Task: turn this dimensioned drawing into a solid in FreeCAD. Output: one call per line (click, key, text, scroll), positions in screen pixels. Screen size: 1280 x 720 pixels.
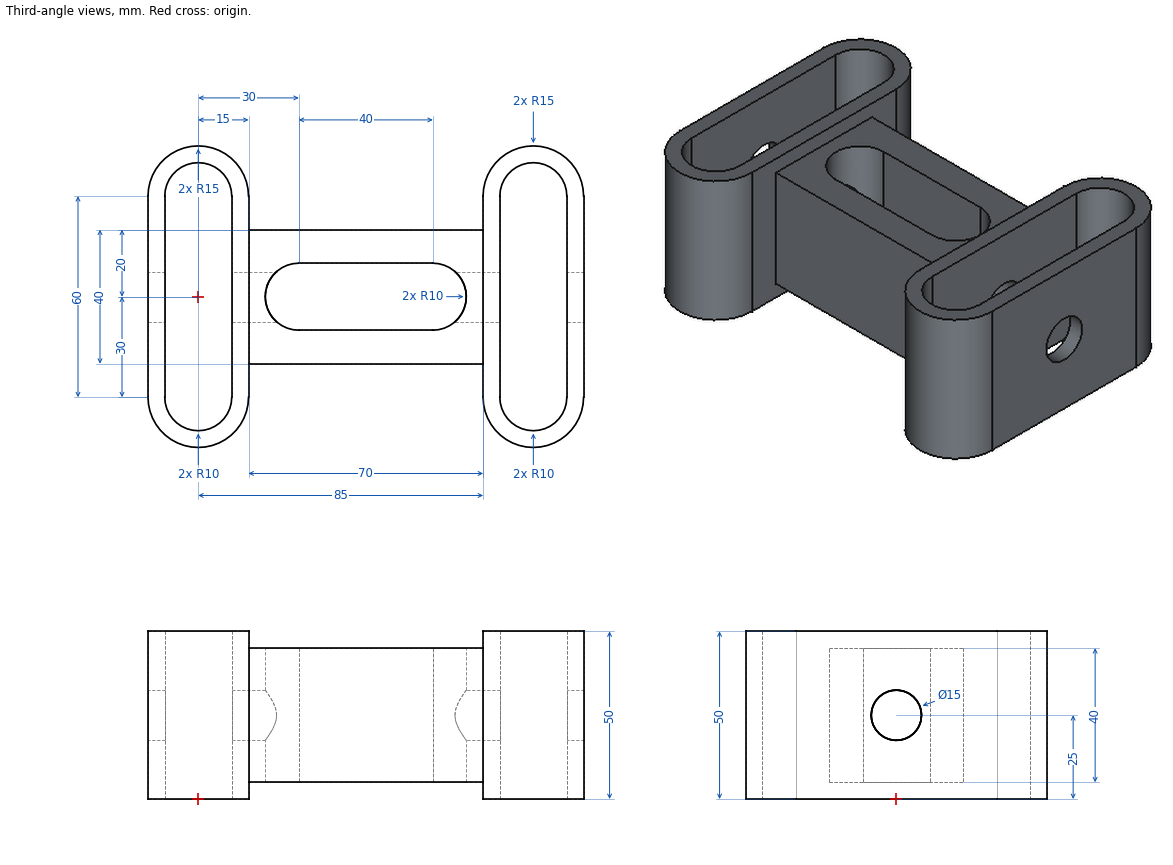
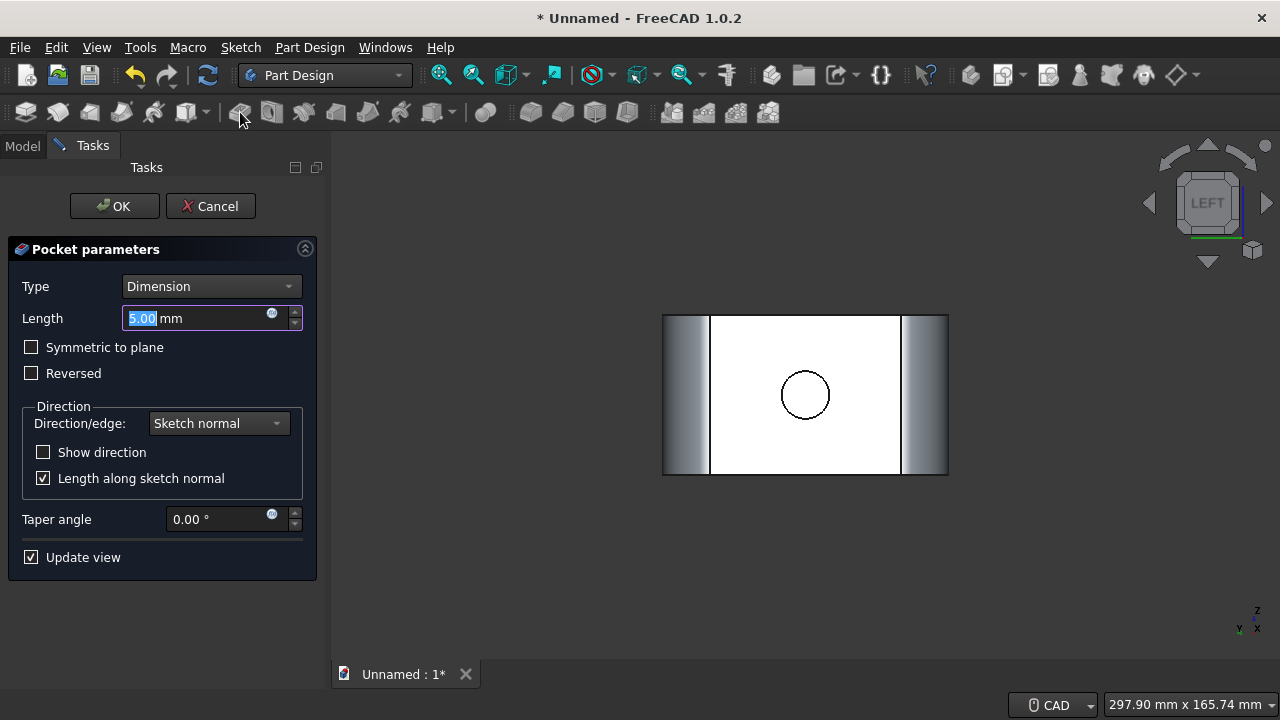
click(212, 286)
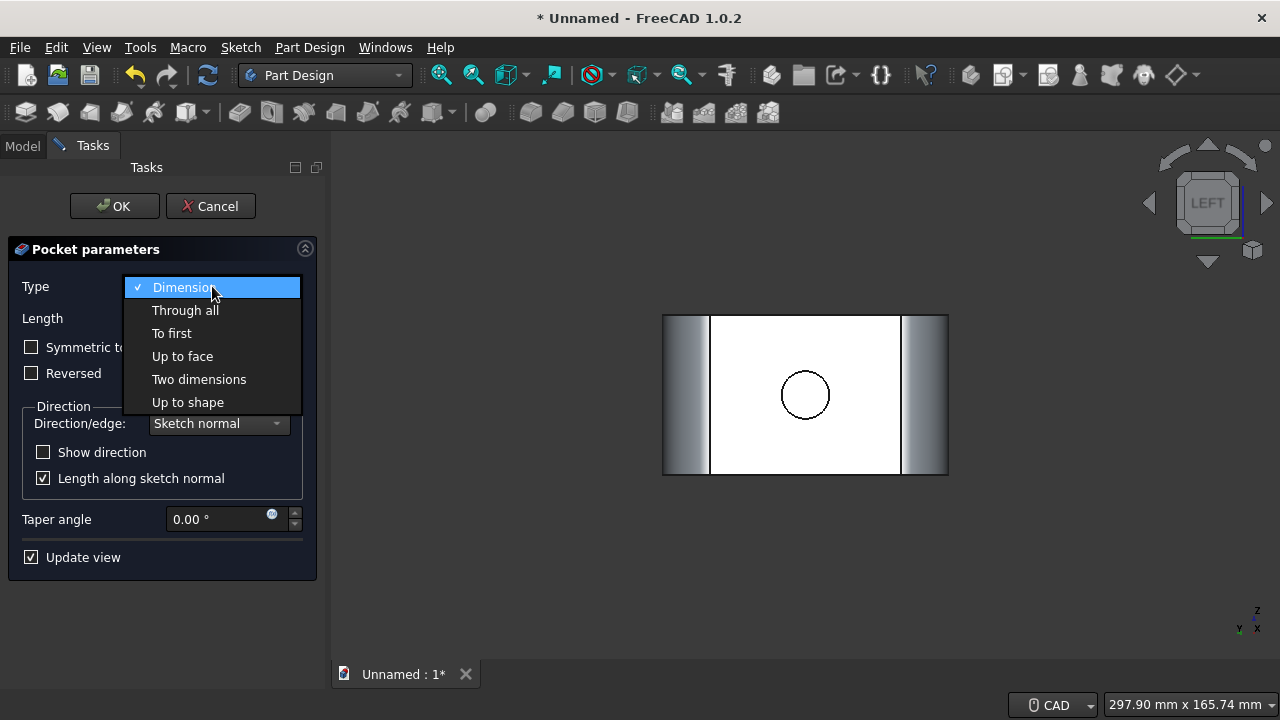
click(212, 310)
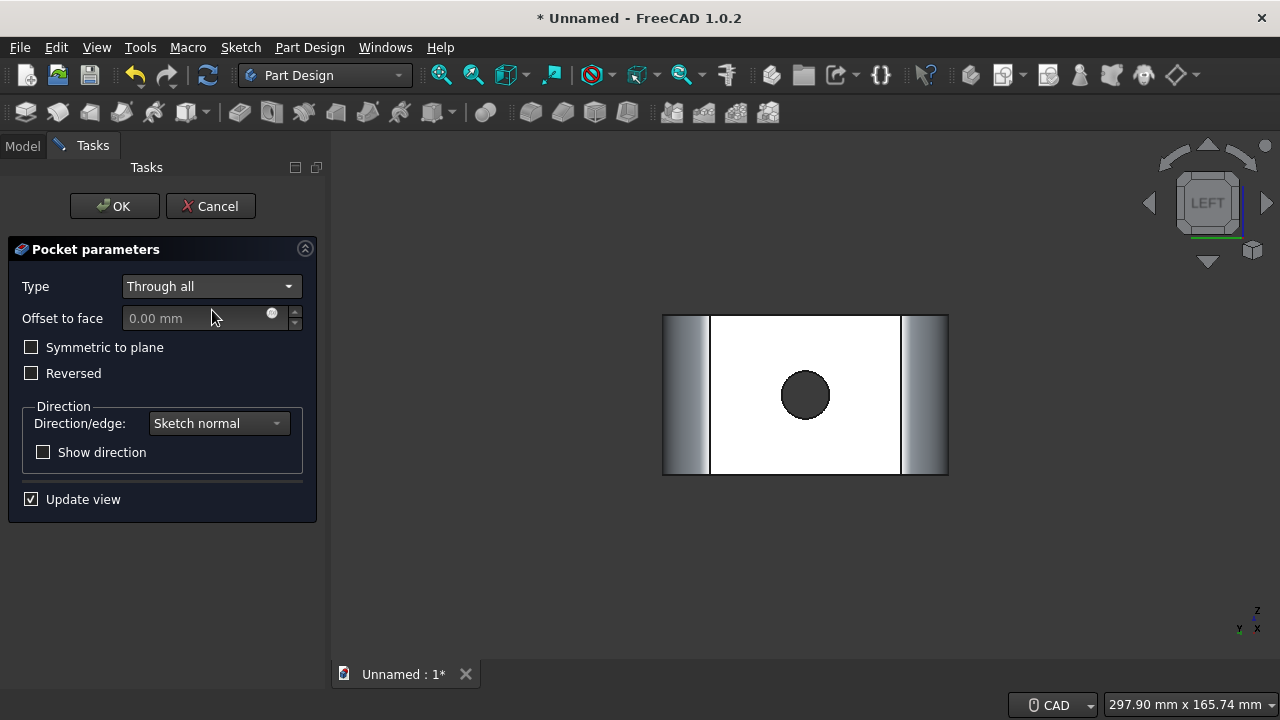
click(115, 206)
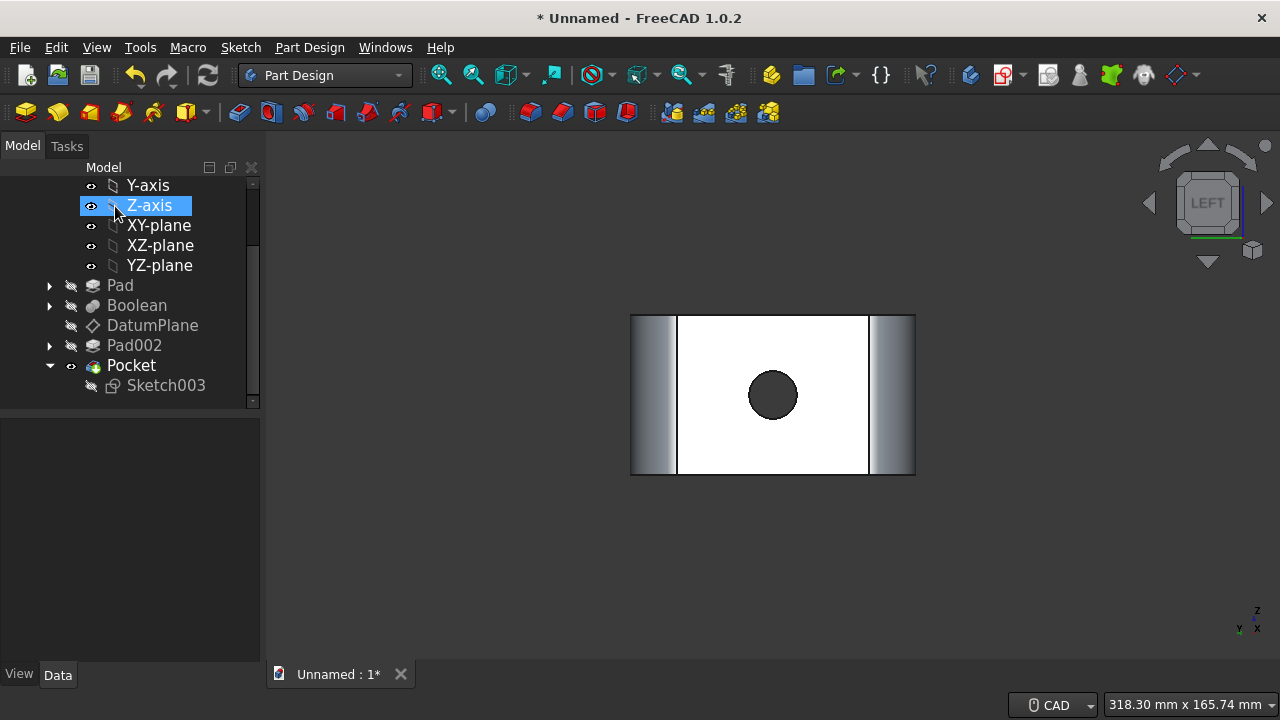
key(0)